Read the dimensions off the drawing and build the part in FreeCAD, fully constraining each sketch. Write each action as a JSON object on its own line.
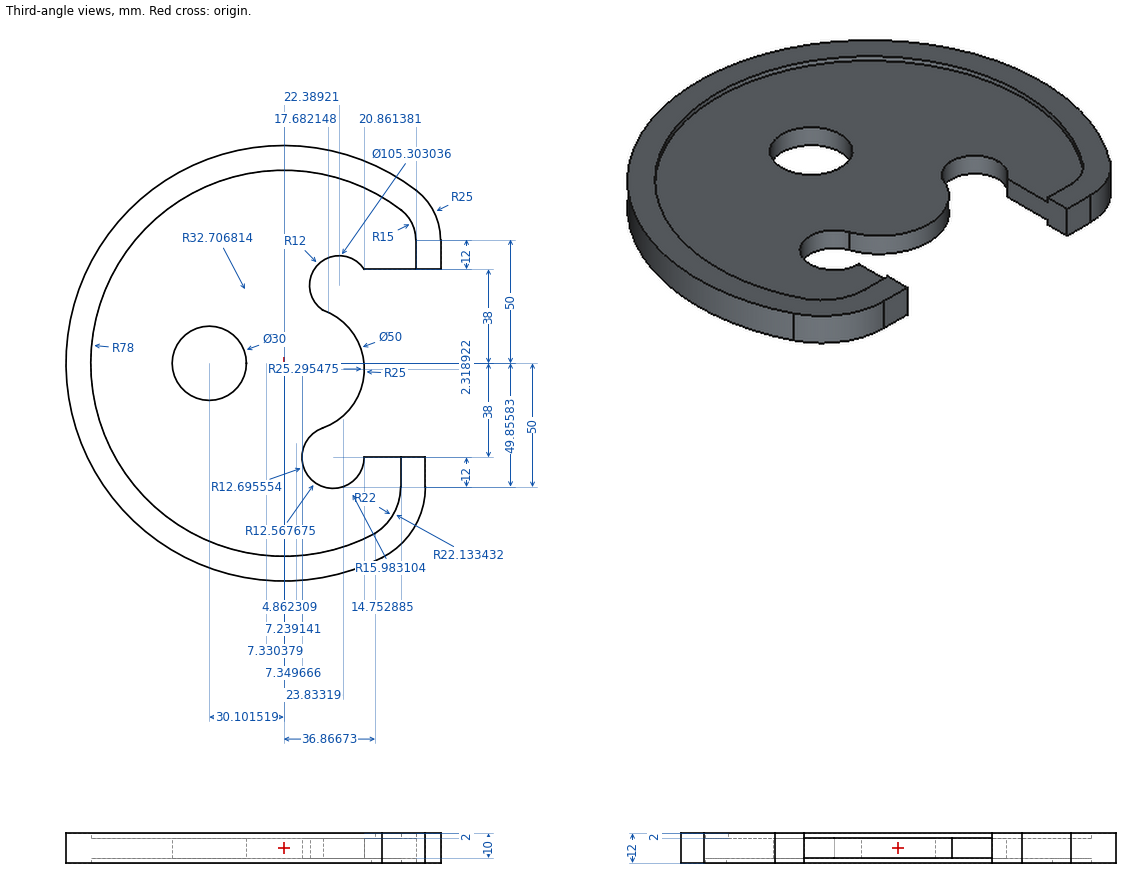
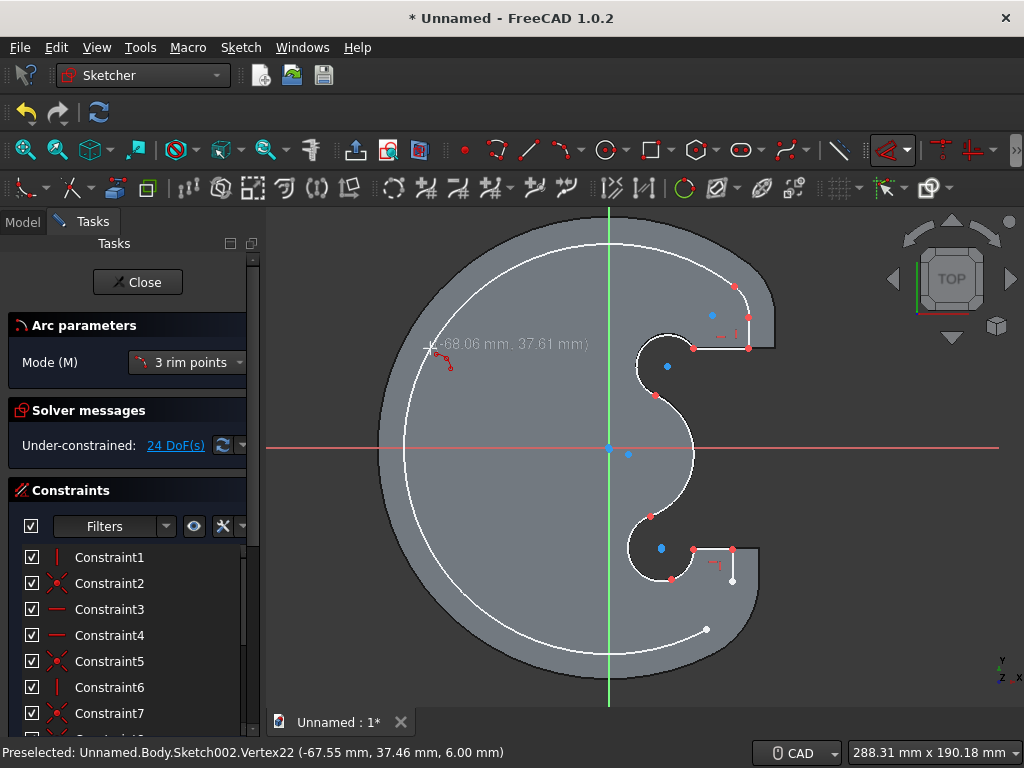
{"action": "left_click", "coordinate": [706, 630]}
{"action": "left_click", "coordinate": [733, 581]}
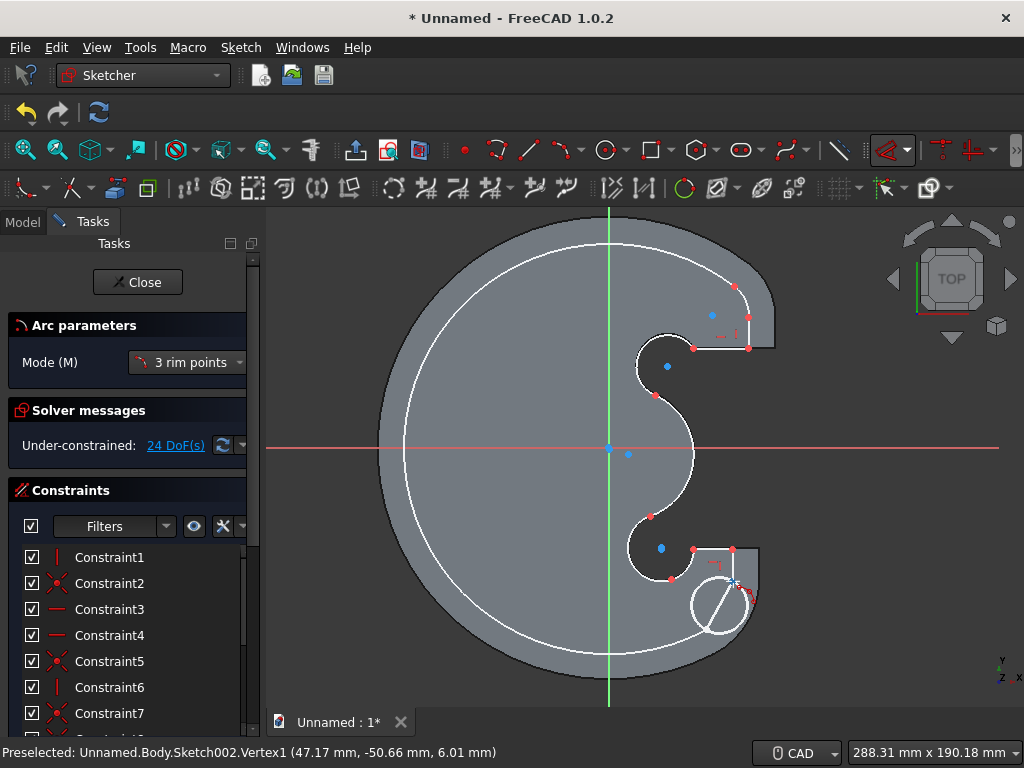
{"action": "scroll", "coordinate": [726, 607], "scroll_direction": "up", "scroll_amount": 4}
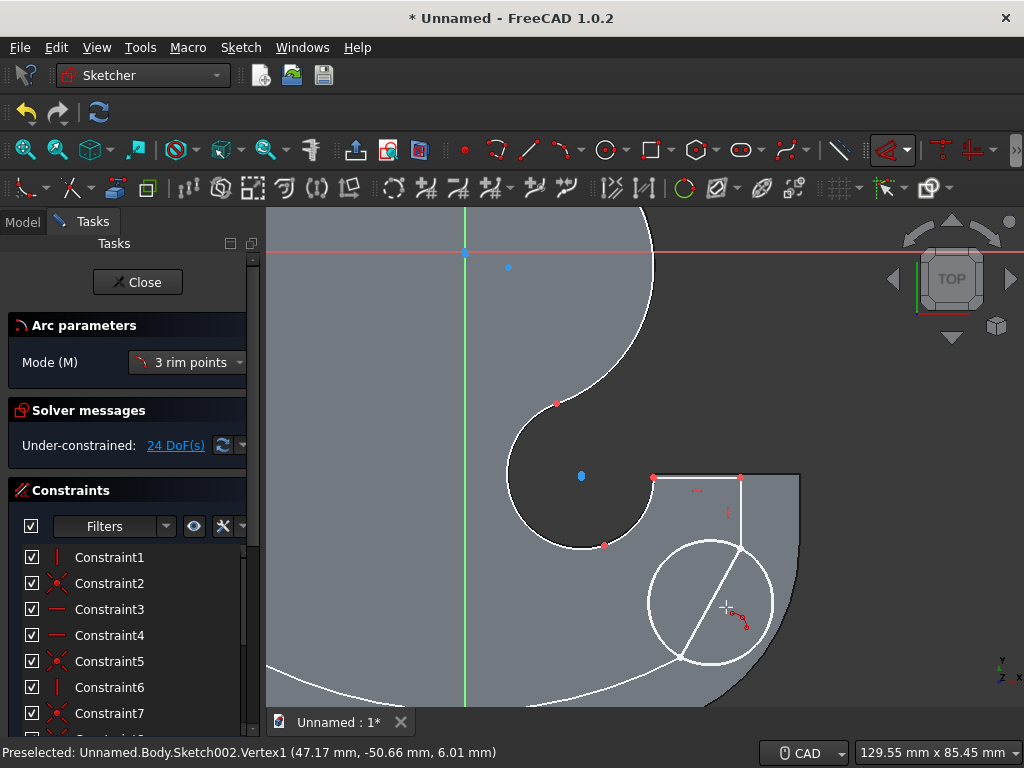
{"action": "left_click", "coordinate": [725, 607]}
{"action": "key", "text": "Escape"}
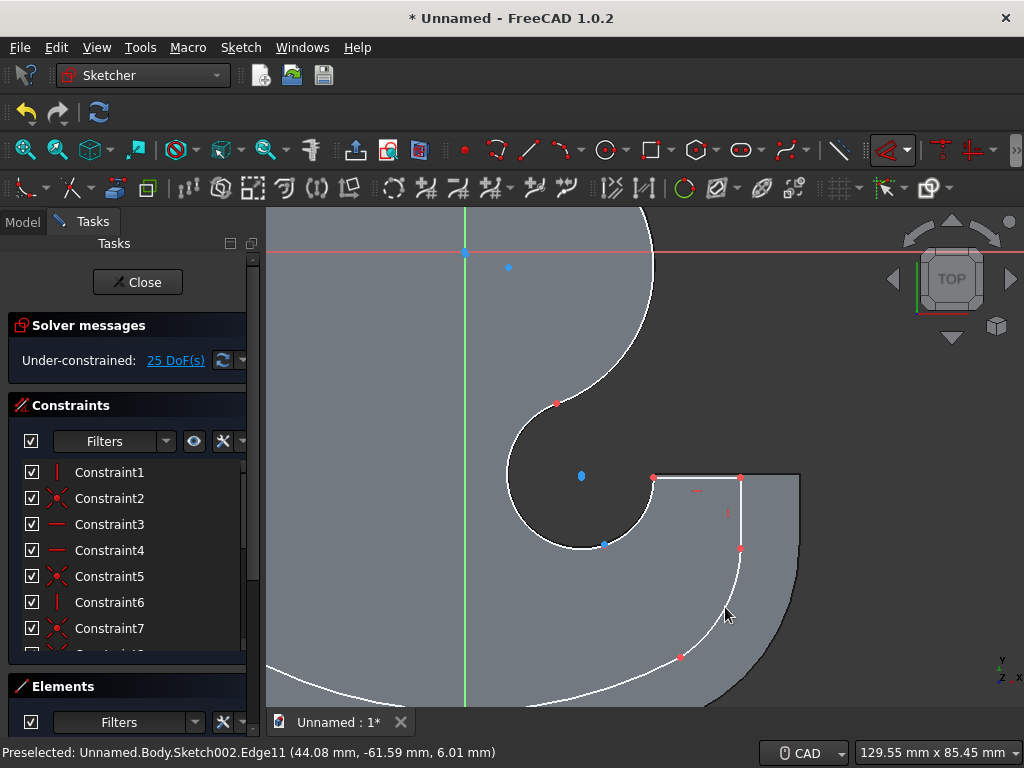
{"action": "left_click", "coordinate": [741, 527]}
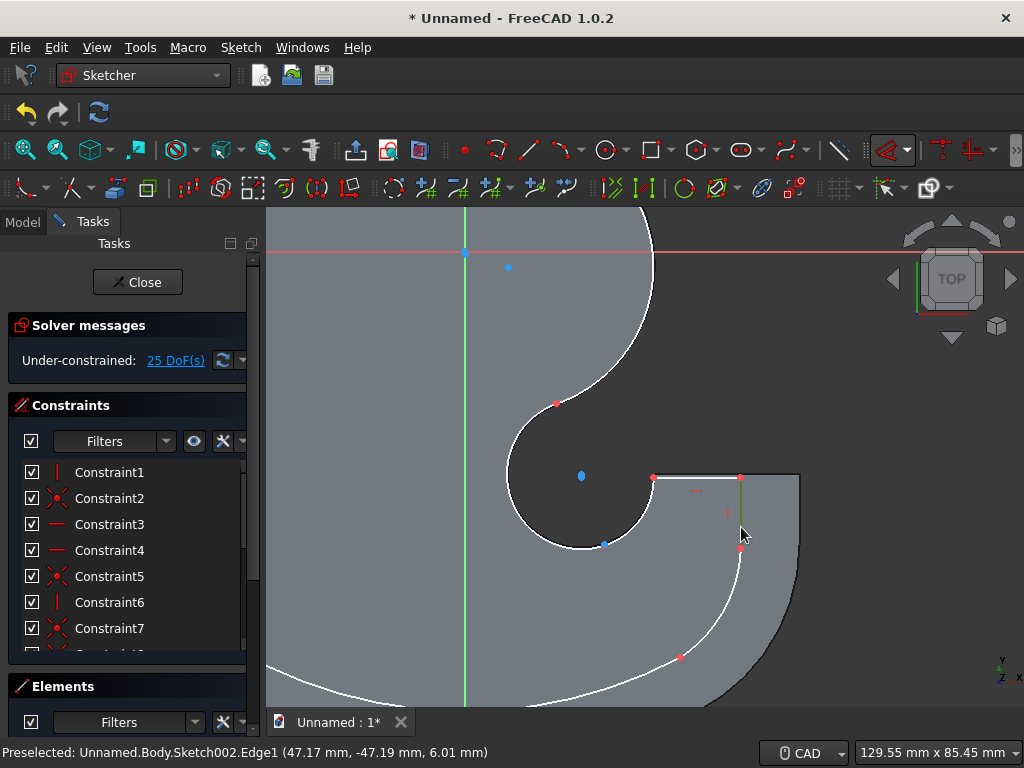
{"action": "left_click", "coordinate": [709, 631]}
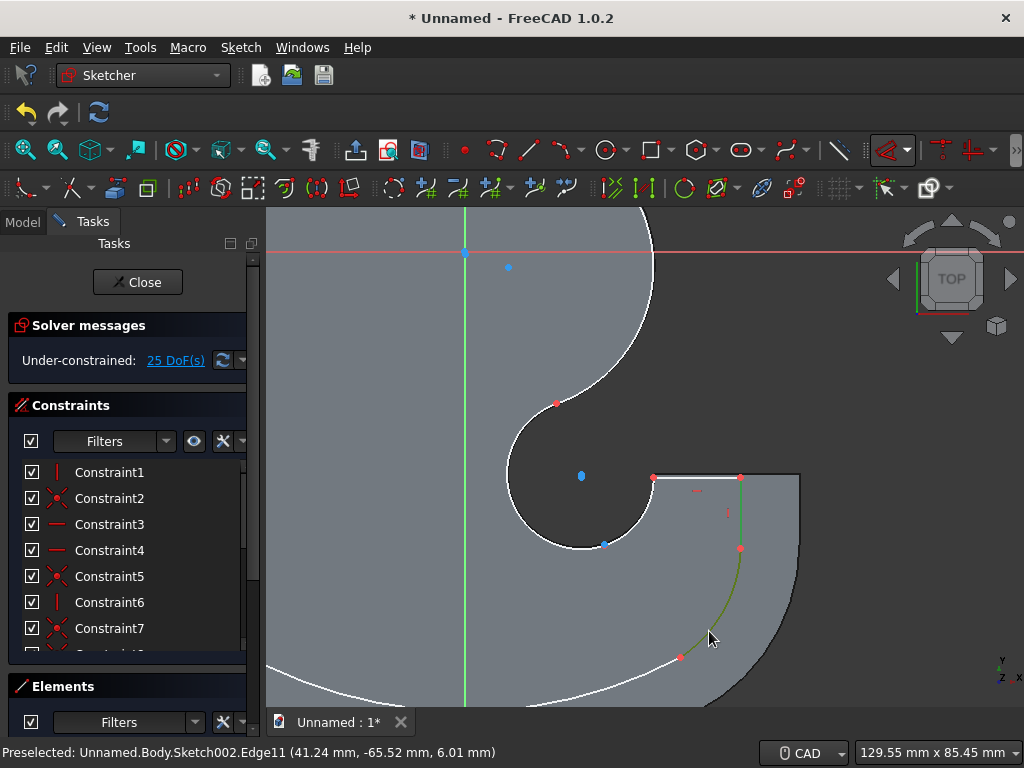
{"action": "key", "text": "t"}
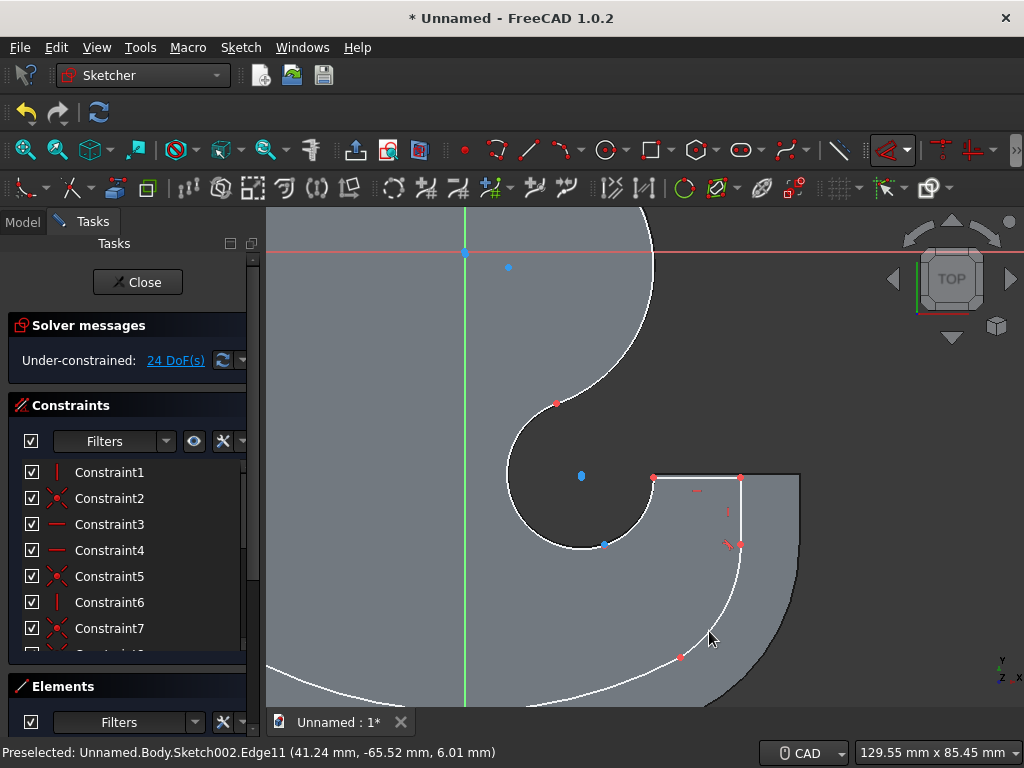
{"action": "scroll", "coordinate": [726, 608], "scroll_direction": "down", "scroll_amount": 4}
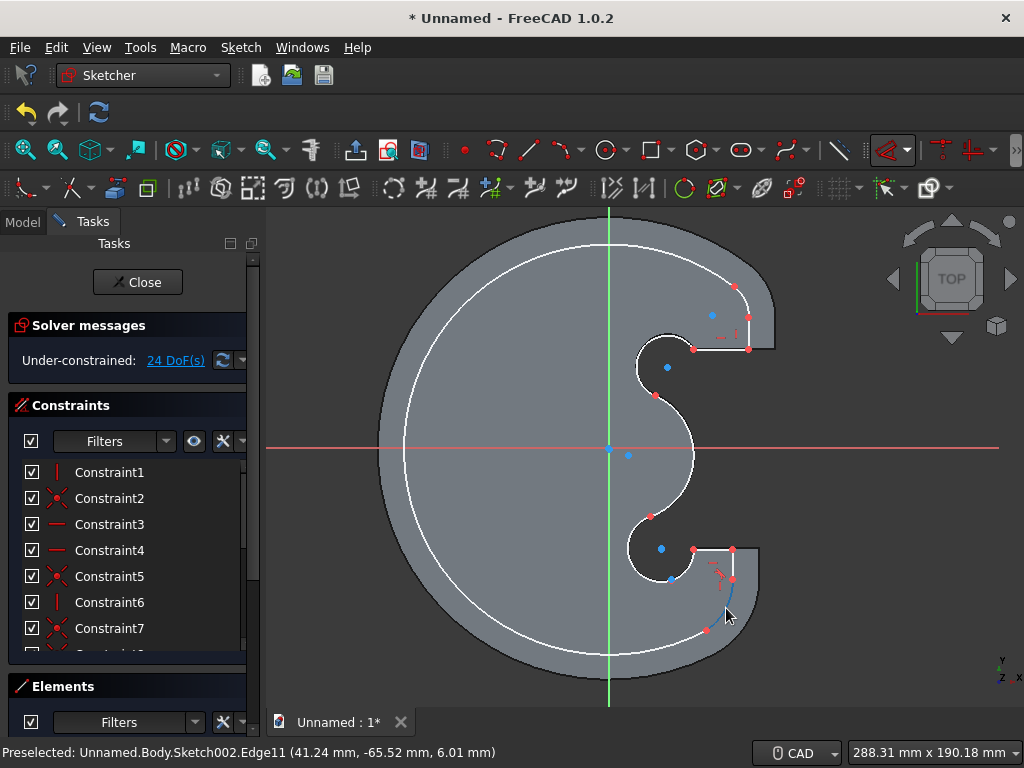
{"action": "scroll", "coordinate": [749, 340], "scroll_direction": "up", "scroll_amount": 2}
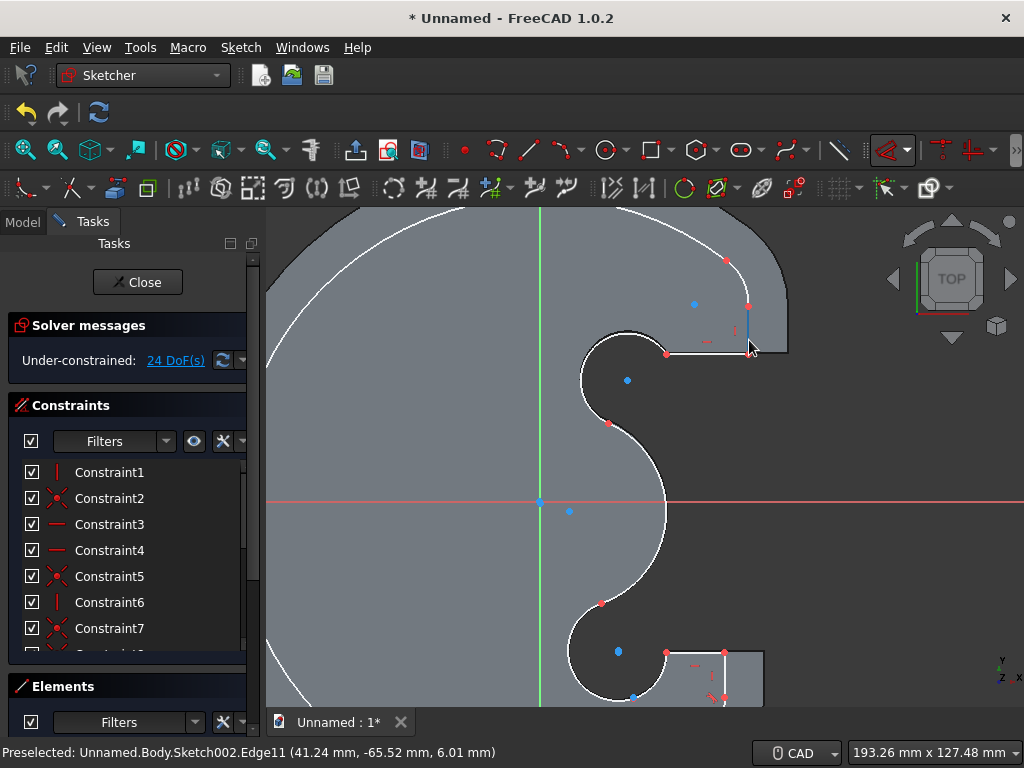
{"action": "left_click", "coordinate": [748, 340]}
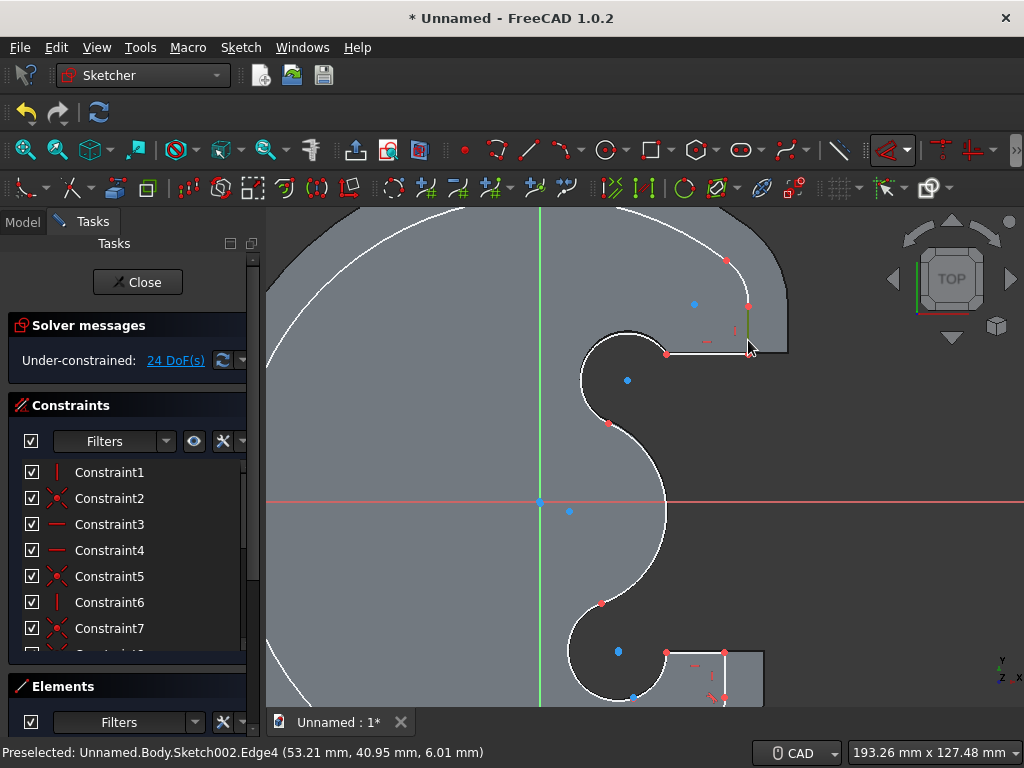
{"action": "left_click", "coordinate": [747, 291]}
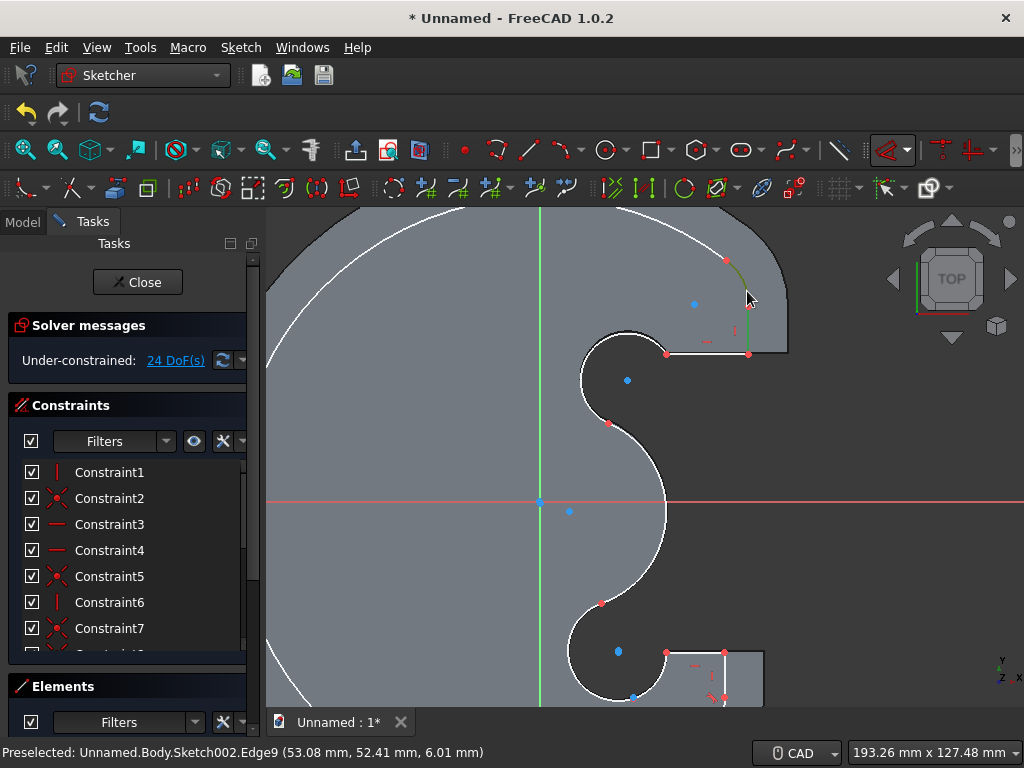
{"action": "key", "text": "t"}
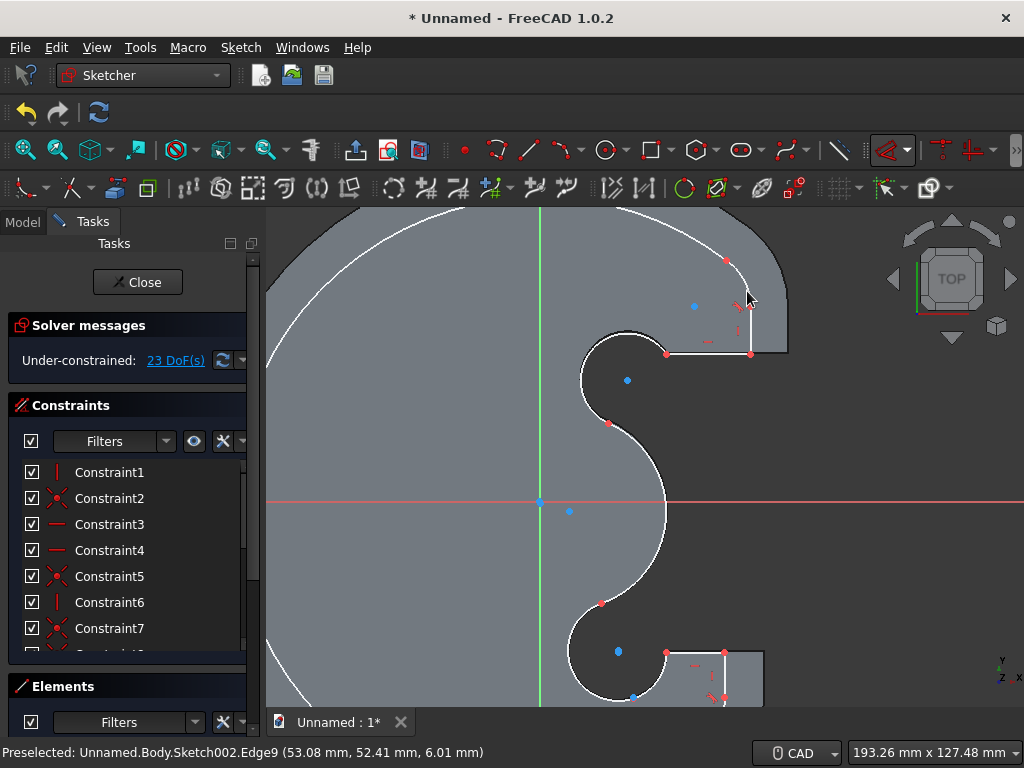
{"action": "left_click", "coordinate": [663, 670]}